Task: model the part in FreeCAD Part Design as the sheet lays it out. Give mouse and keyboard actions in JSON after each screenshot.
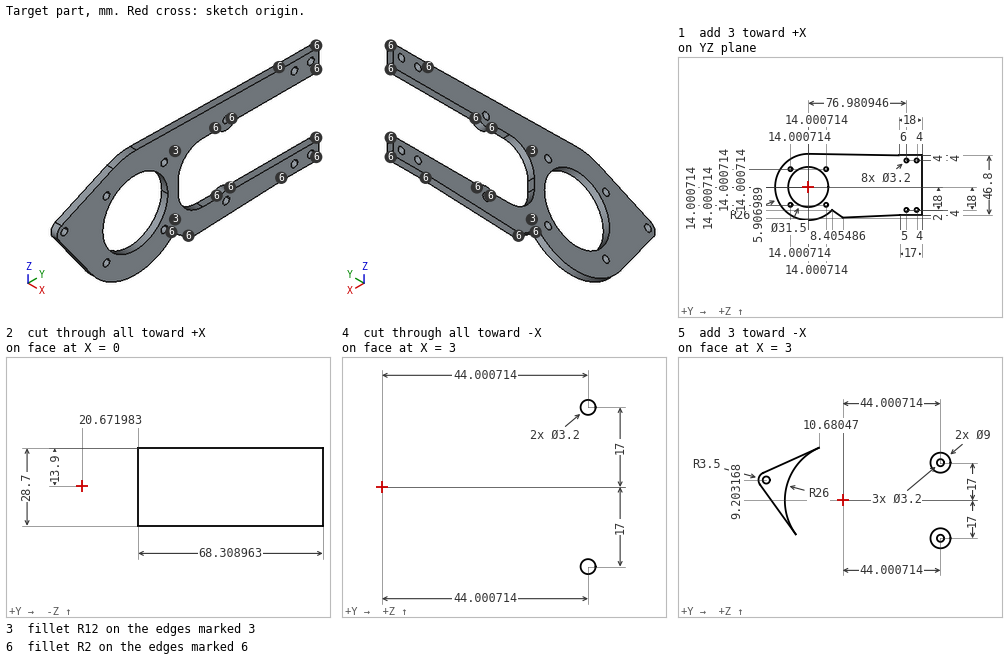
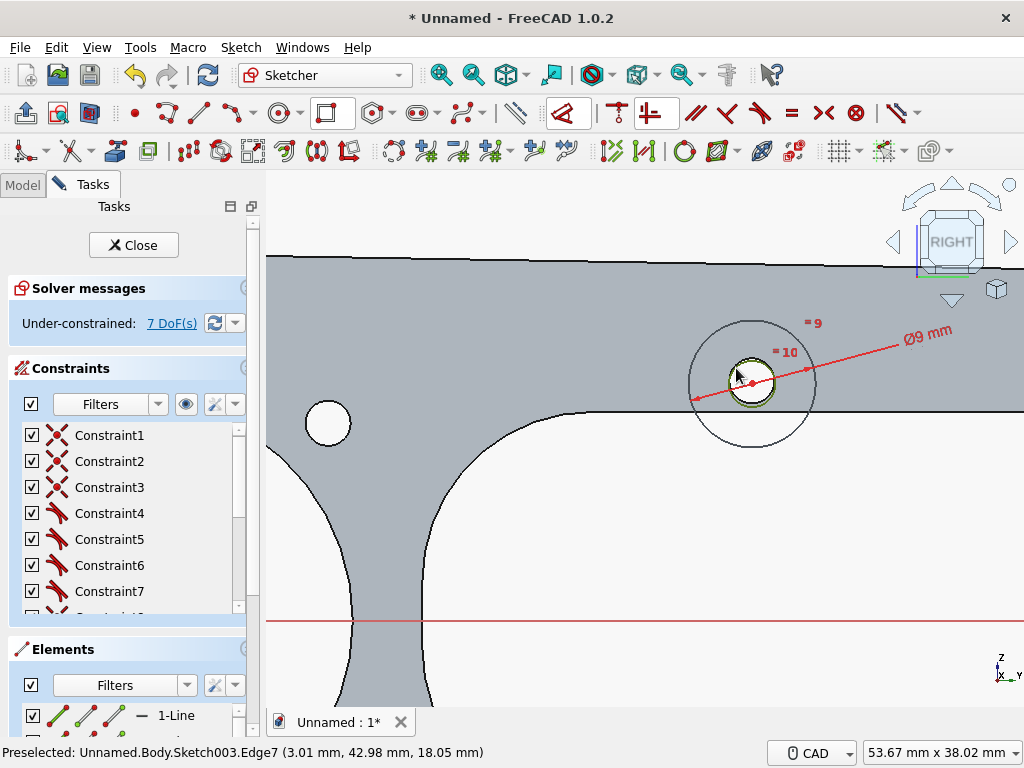
{"action": "key", "text": "k o"}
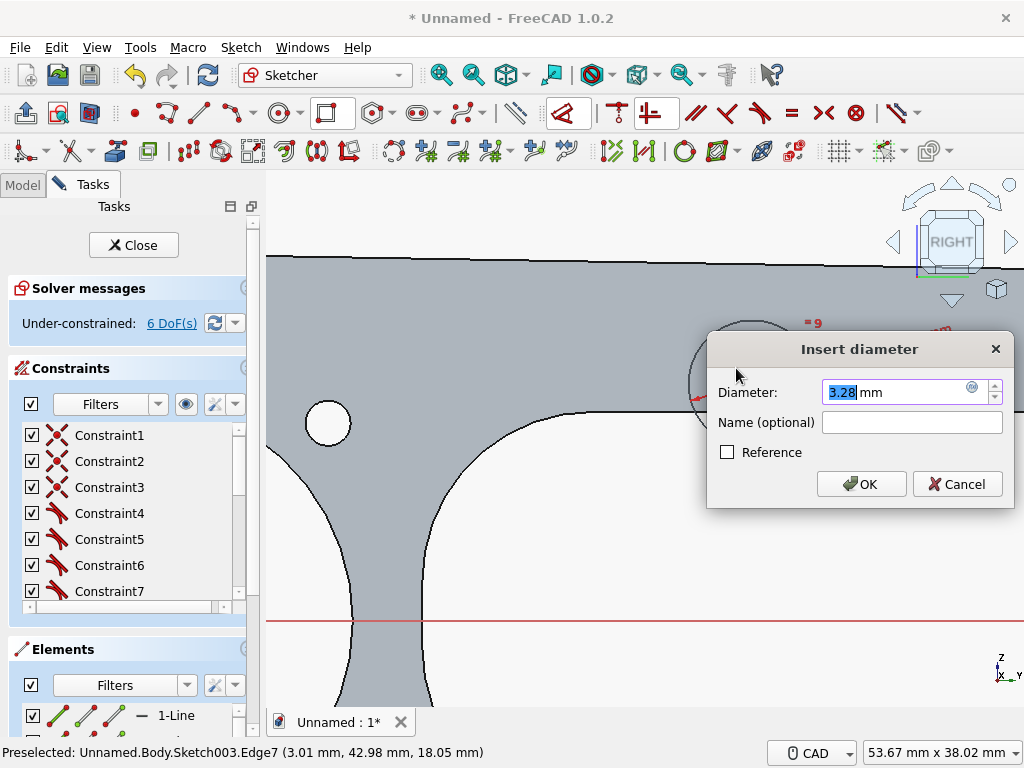
{"action": "type", "text": "3.2"}
{"action": "key", "text": "Return"}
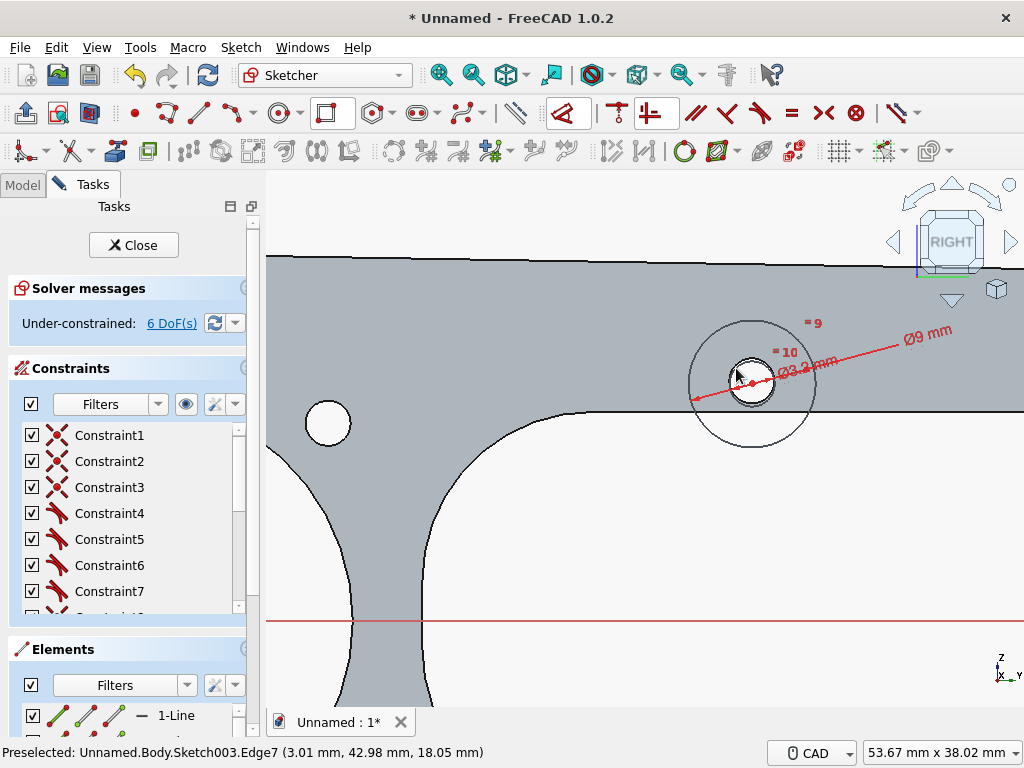
{"action": "left_click", "coordinate": [752, 384]}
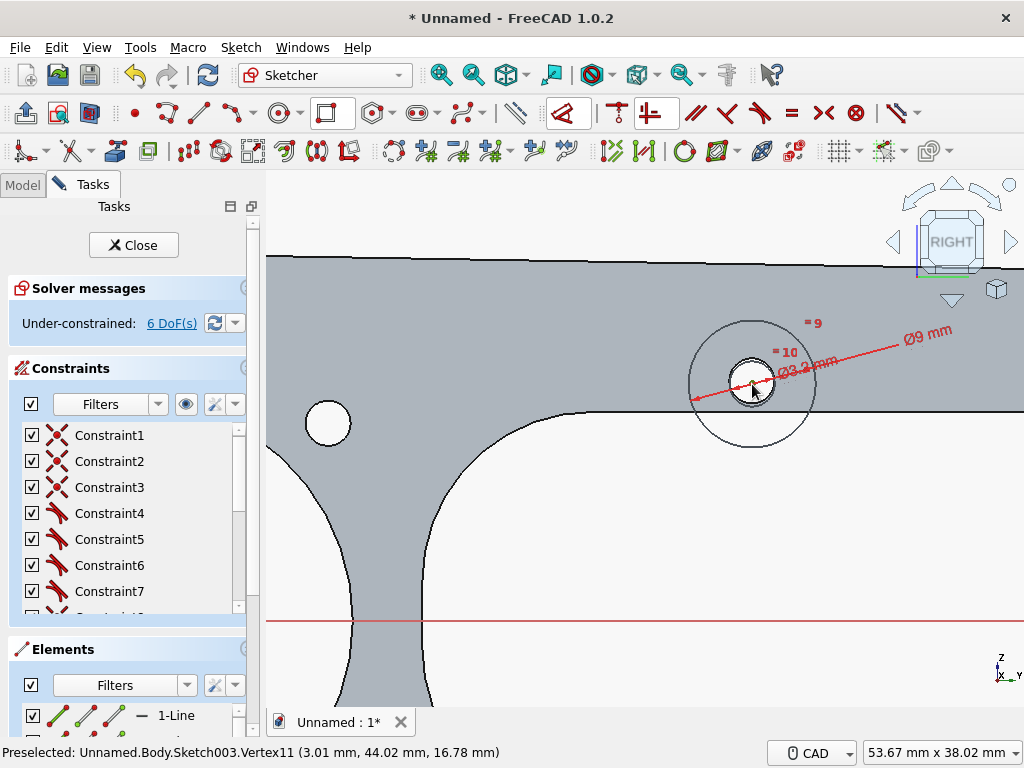
{"action": "left_click", "coordinate": [586, 114]}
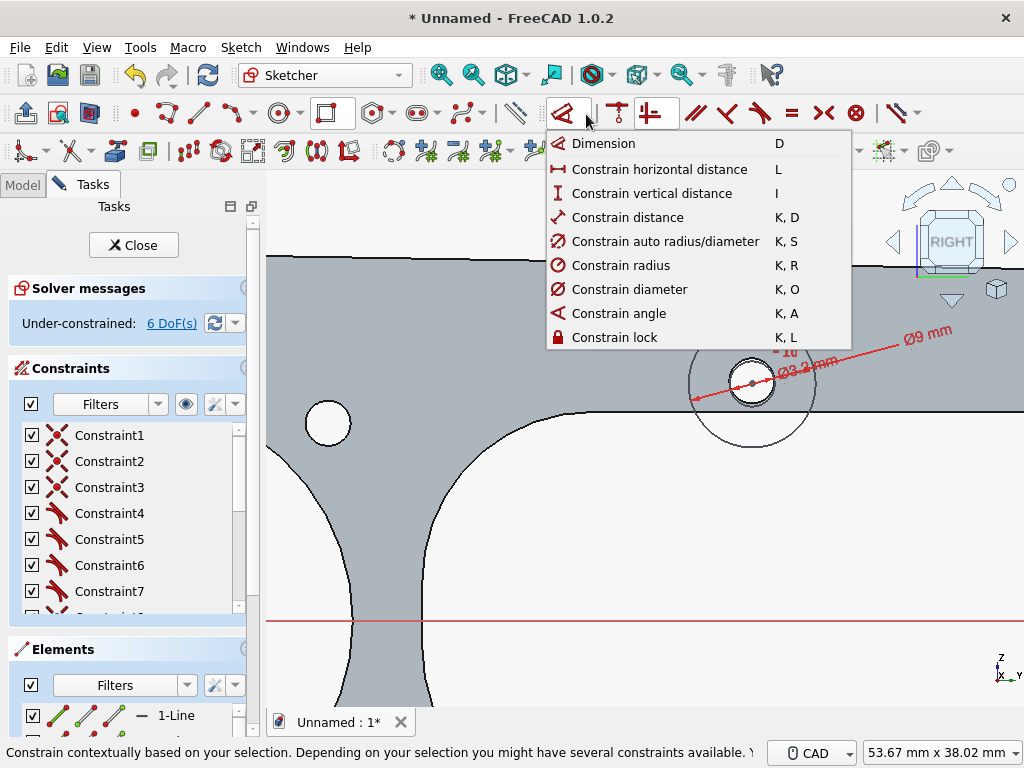
{"action": "left_click", "coordinate": [699, 193]}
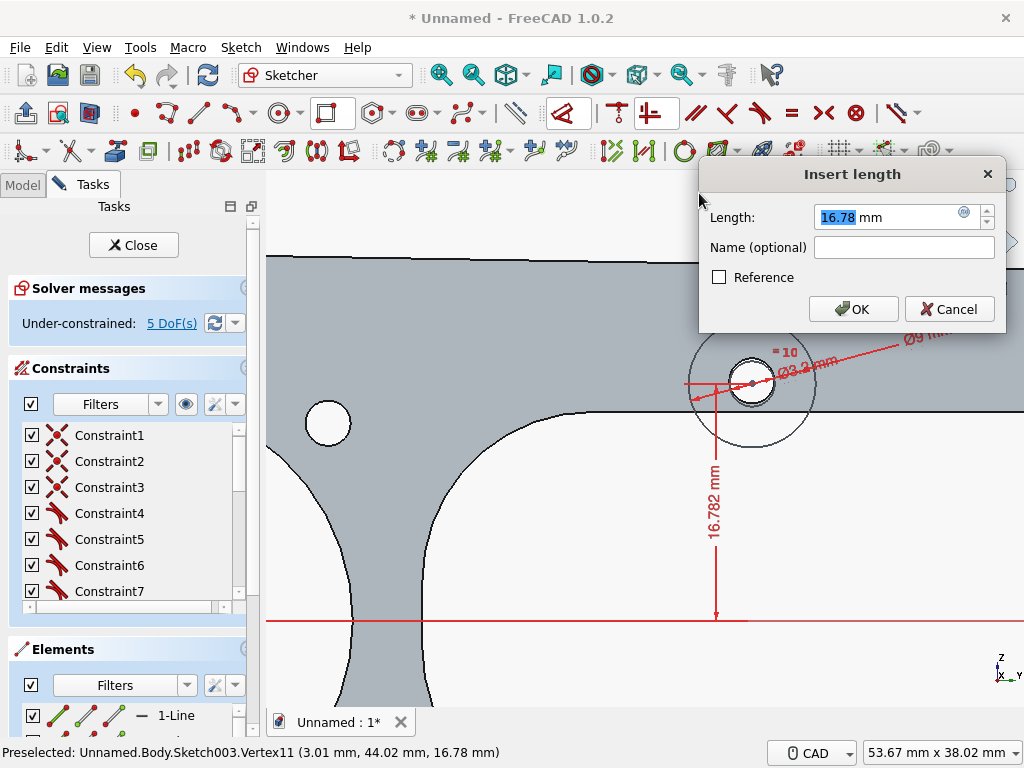
{"action": "type", "text": "17"}
{"action": "key", "text": "Return"}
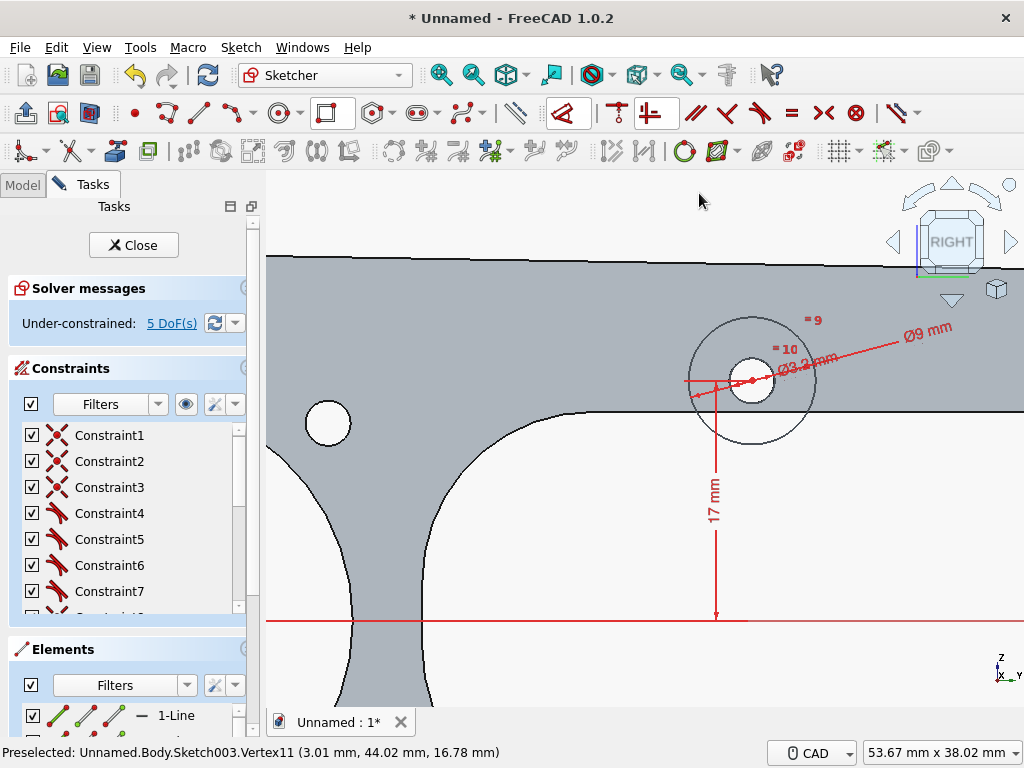
{"action": "scroll", "coordinate": [736, 367], "scroll_direction": "down", "scroll_amount": 6}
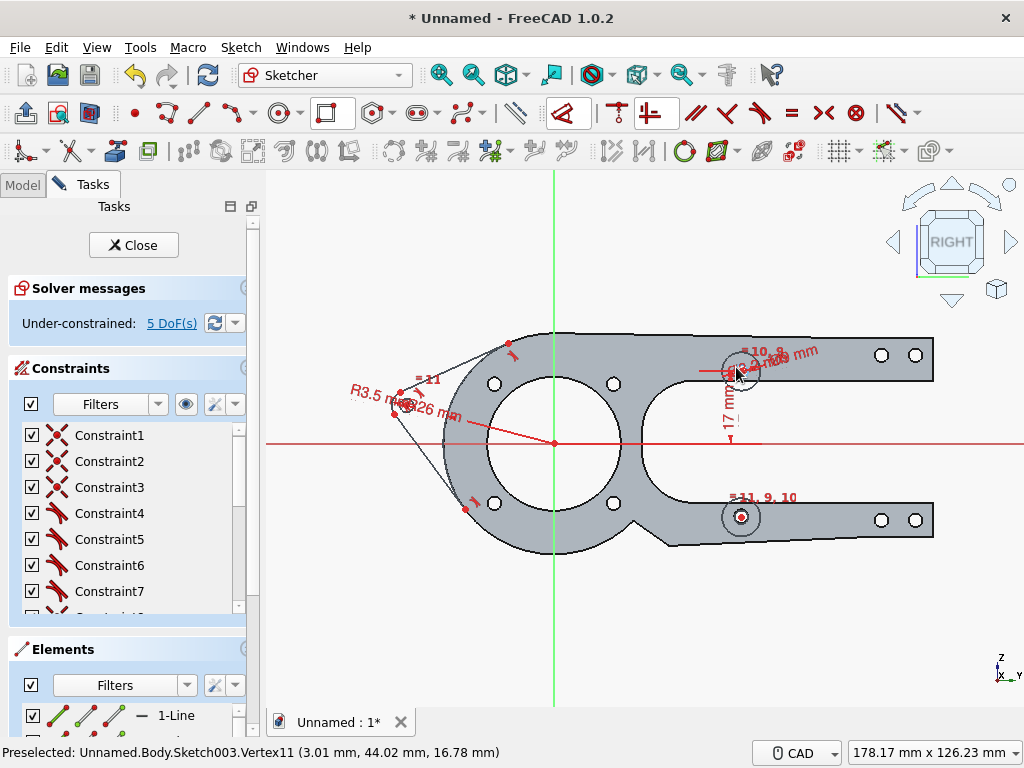
{"action": "left_click", "coordinate": [741, 517]}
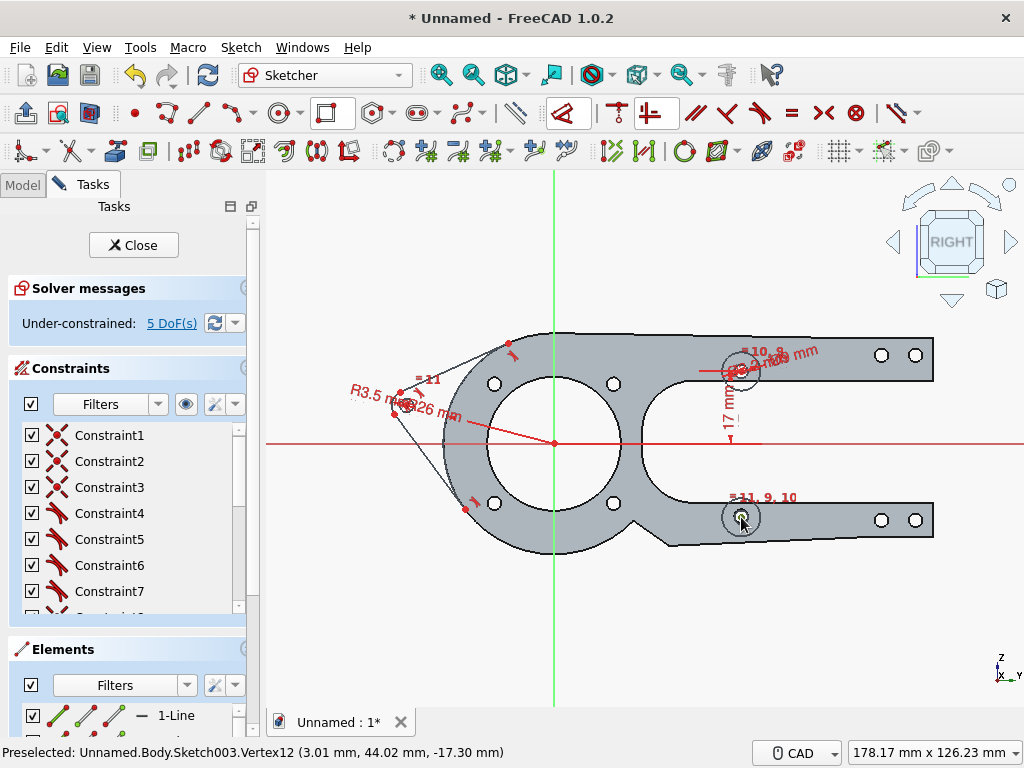
{"action": "key", "text": "i"}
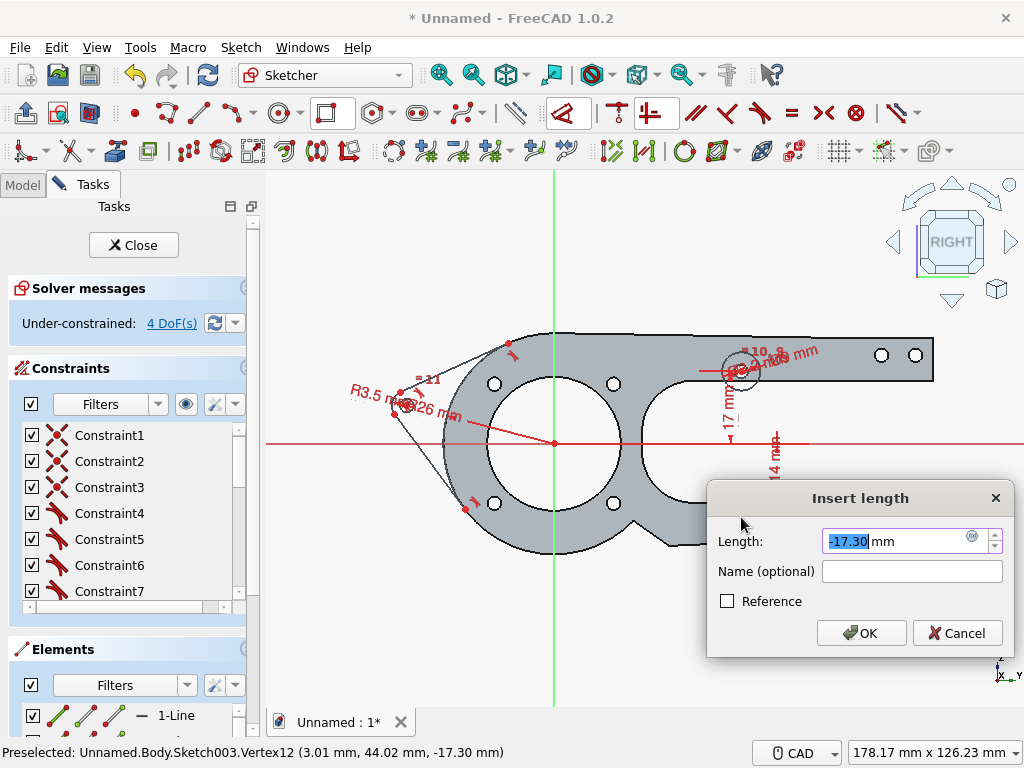
{"action": "type", "text": "-17"}
{"action": "key", "text": "Return"}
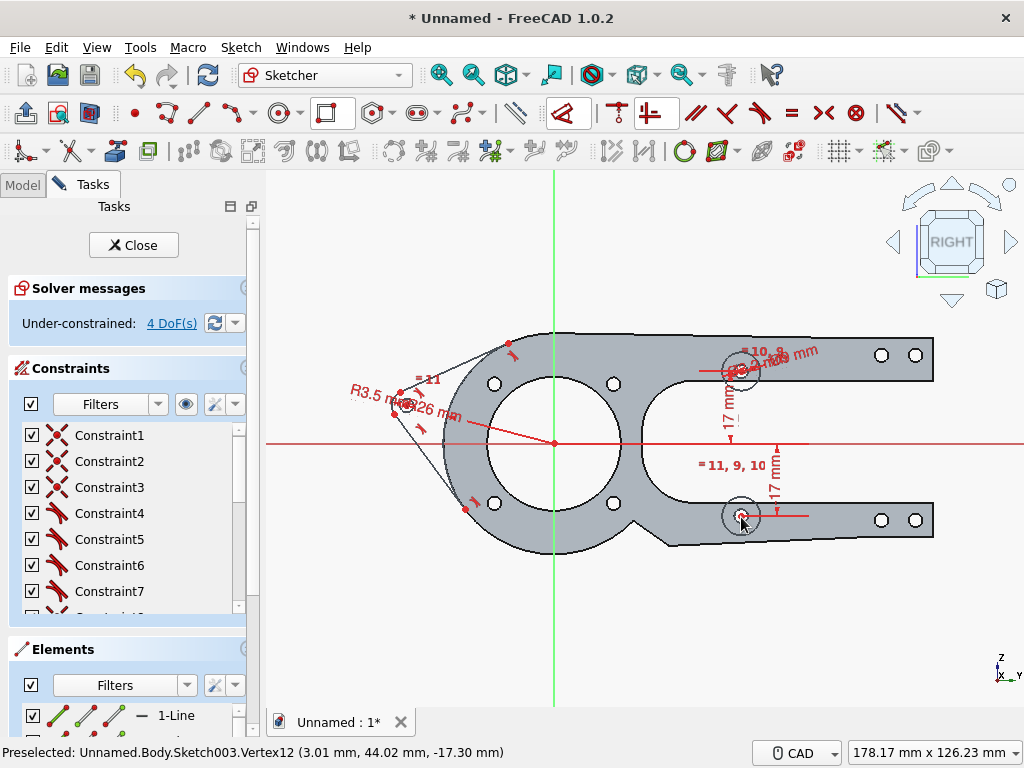
{"action": "left_click", "coordinate": [407, 406]}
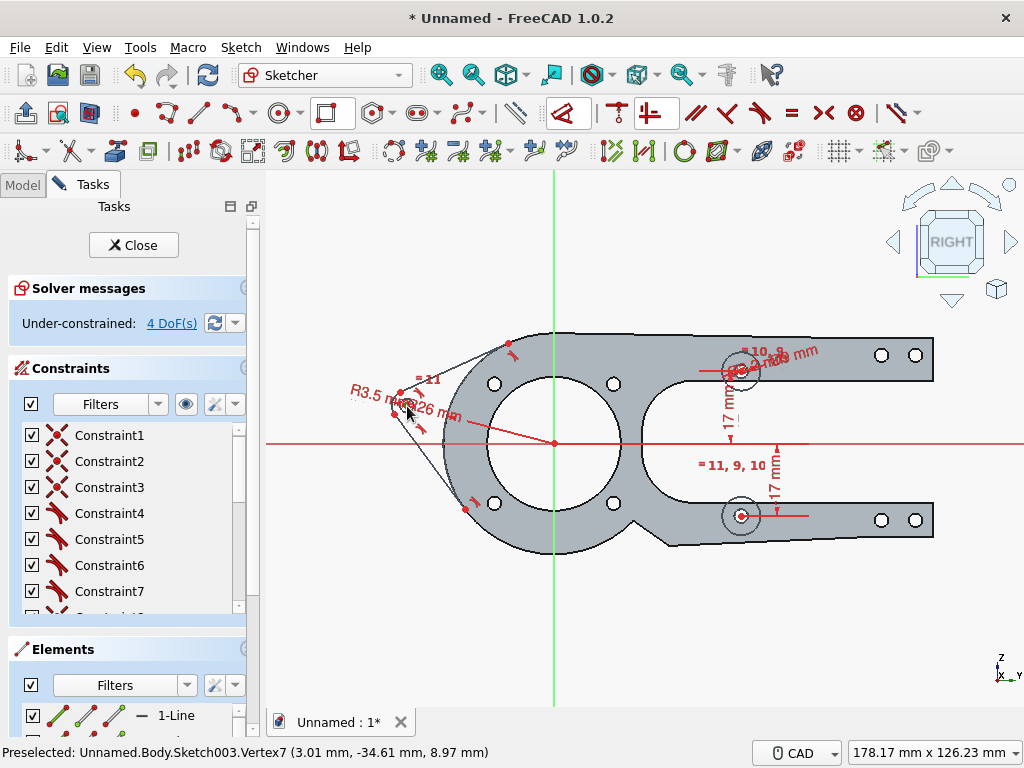
{"action": "key", "text": "i"}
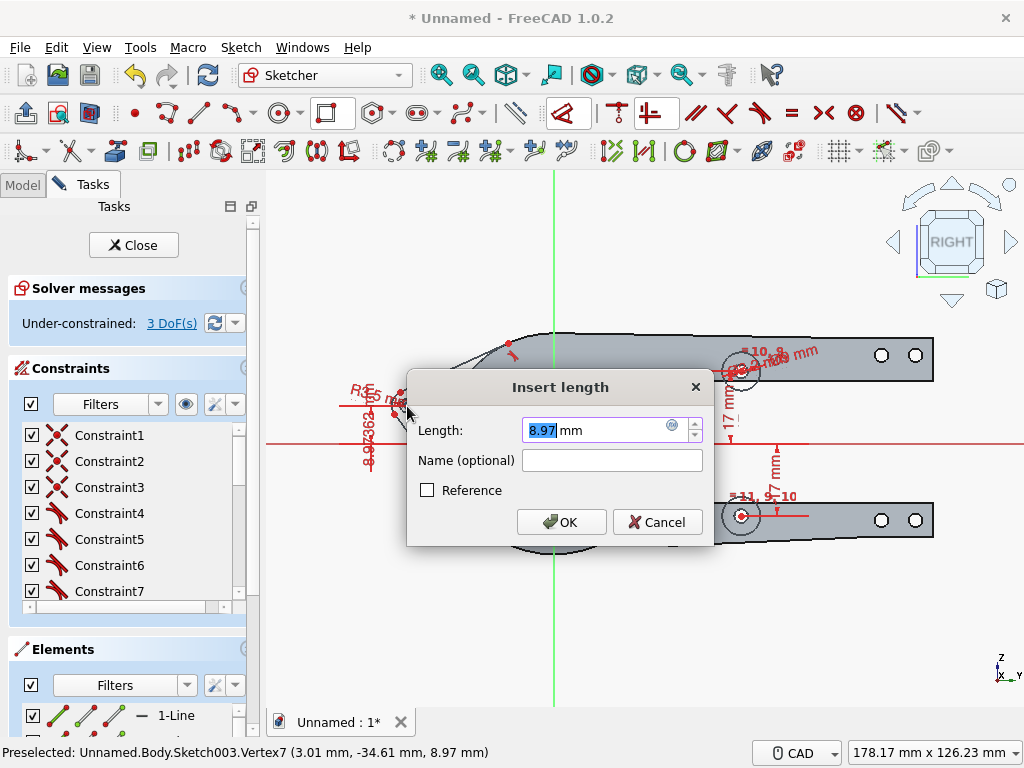
{"action": "type", "text": "9.203168"}
{"action": "key", "text": "Return"}